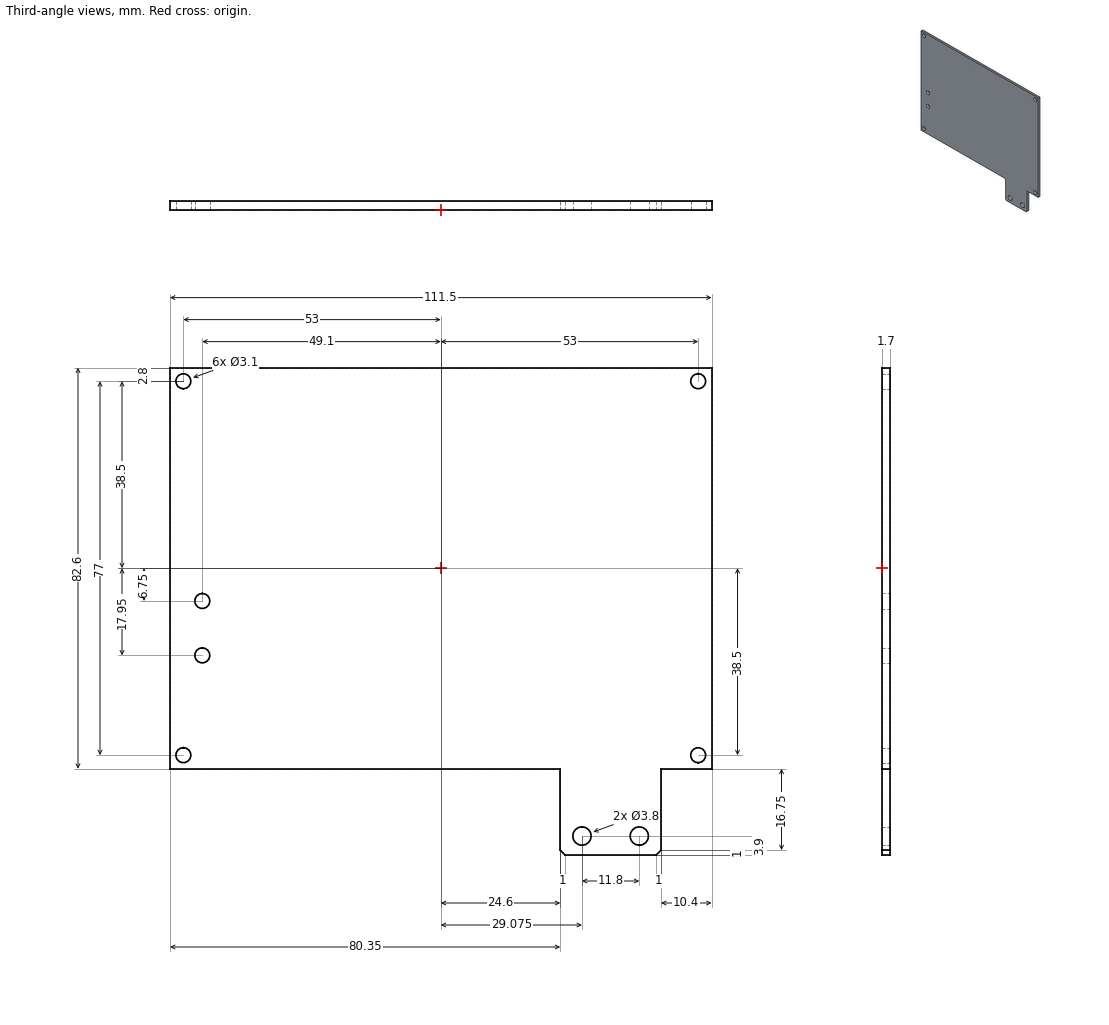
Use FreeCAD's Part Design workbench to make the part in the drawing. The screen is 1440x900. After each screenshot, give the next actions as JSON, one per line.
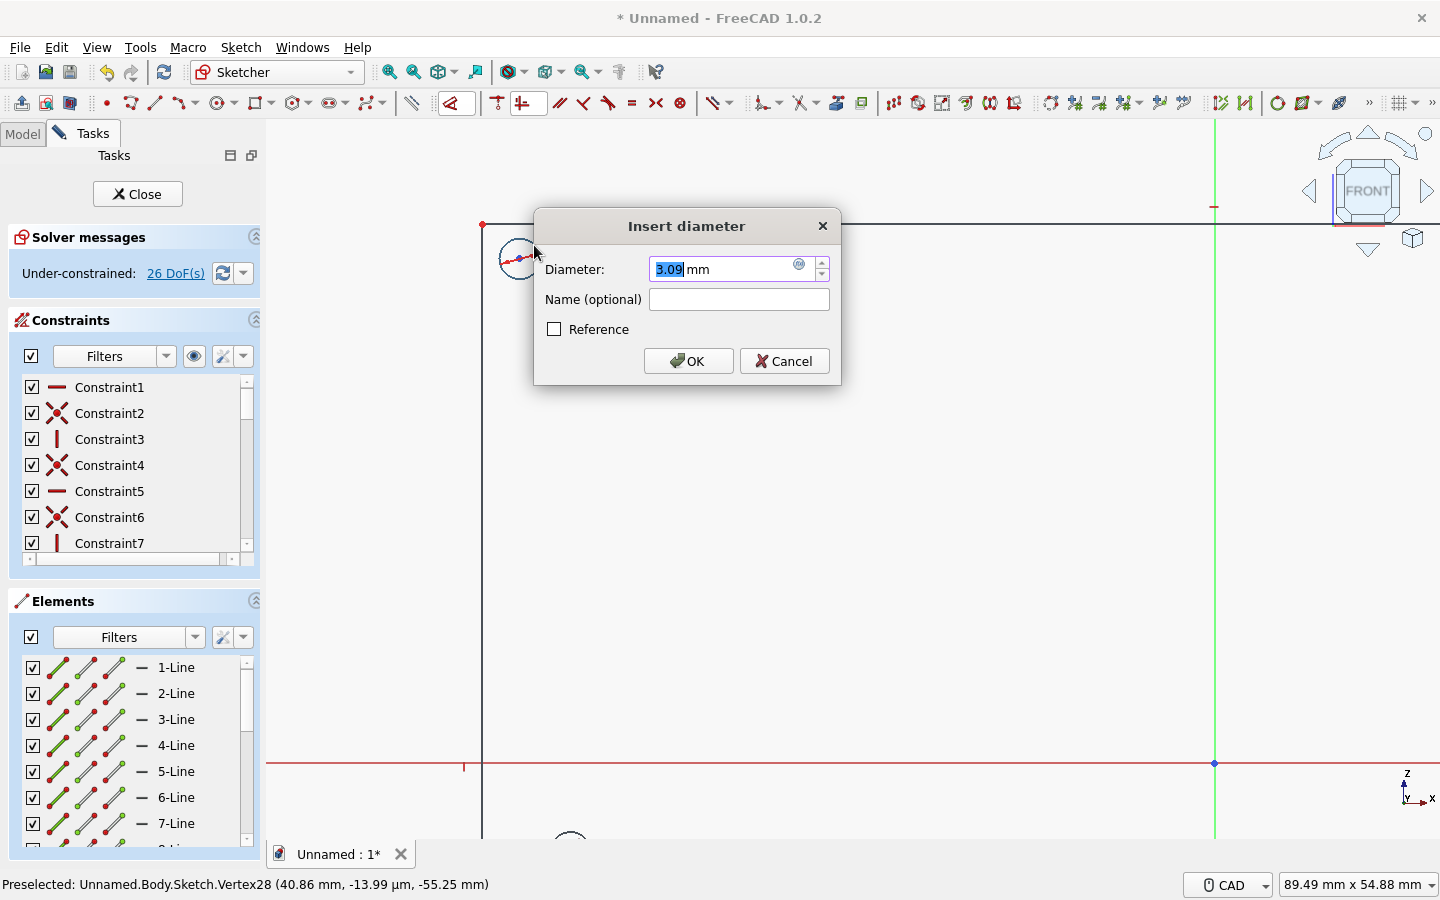
{"action": "type", "text": "3.1"}
{"action": "key", "text": "Return"}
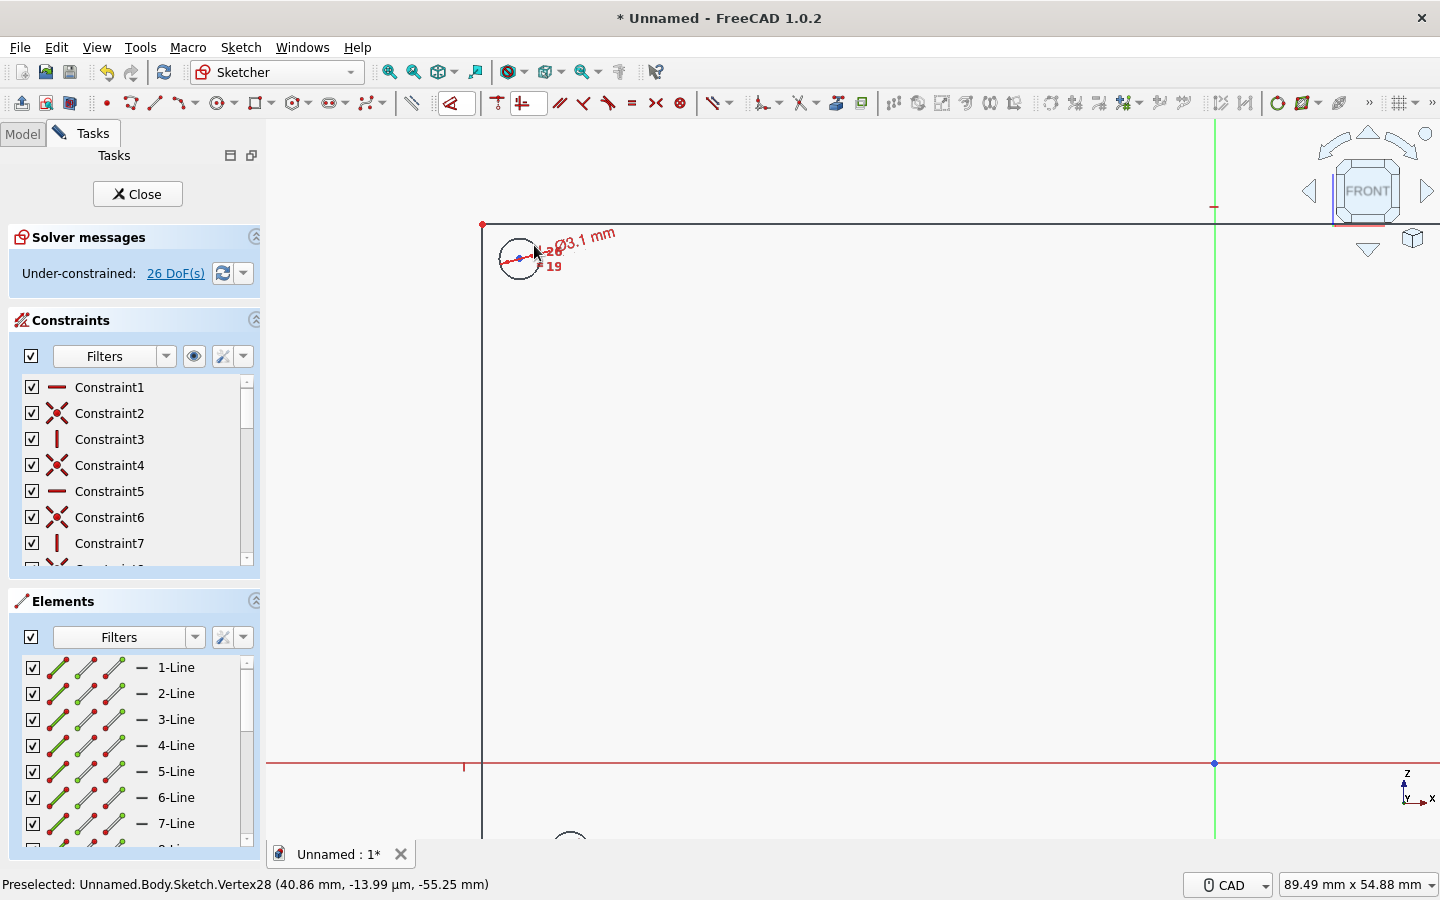
{"action": "scroll", "coordinate": [534, 246], "scroll_direction": "down", "scroll_amount": 5}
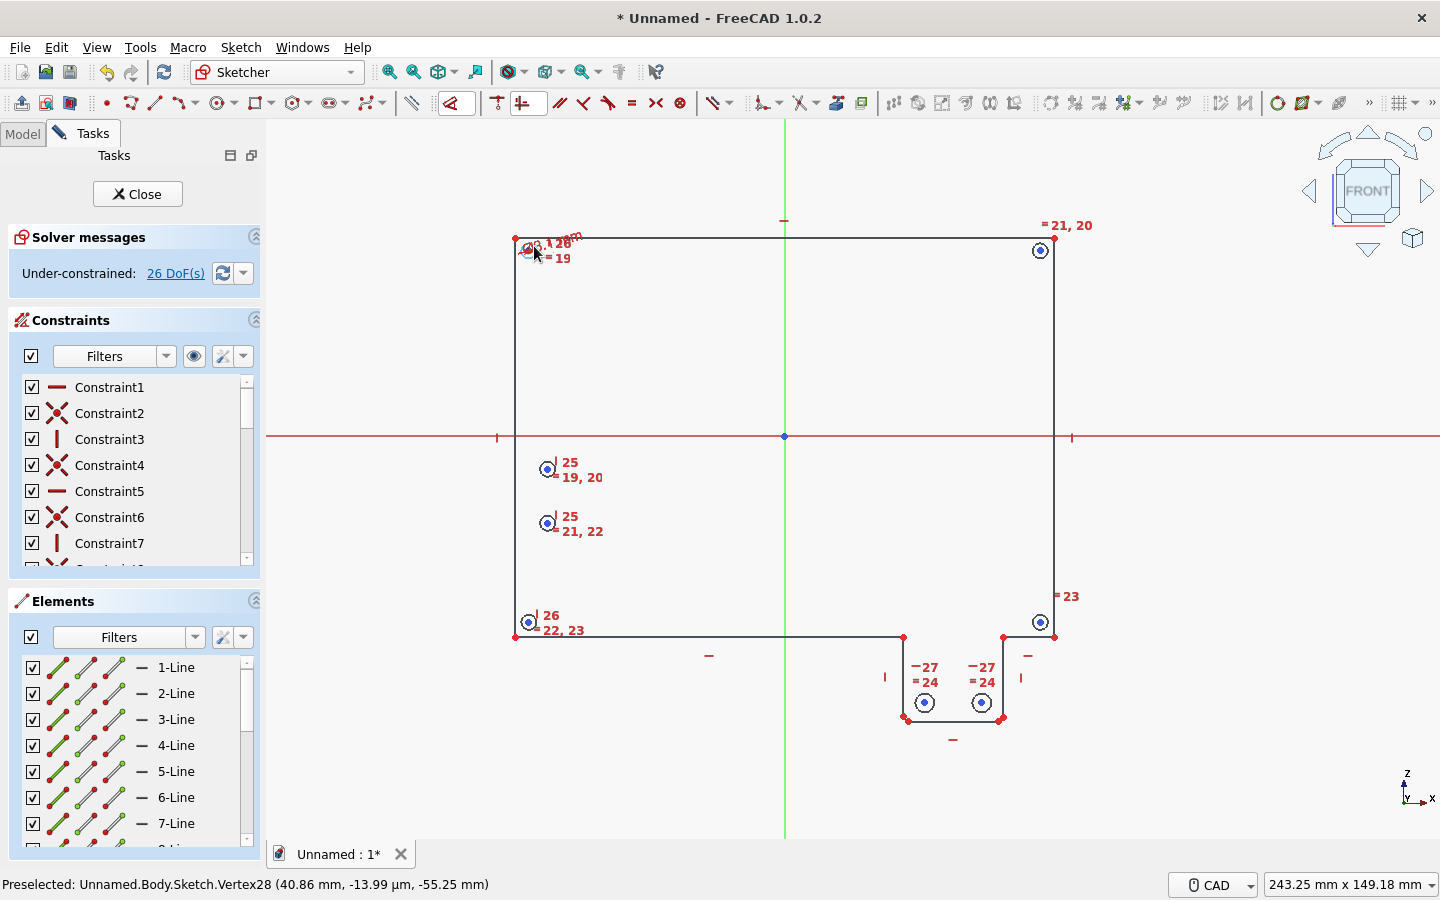
{"action": "scroll", "coordinate": [931, 696], "scroll_direction": "up", "scroll_amount": 4}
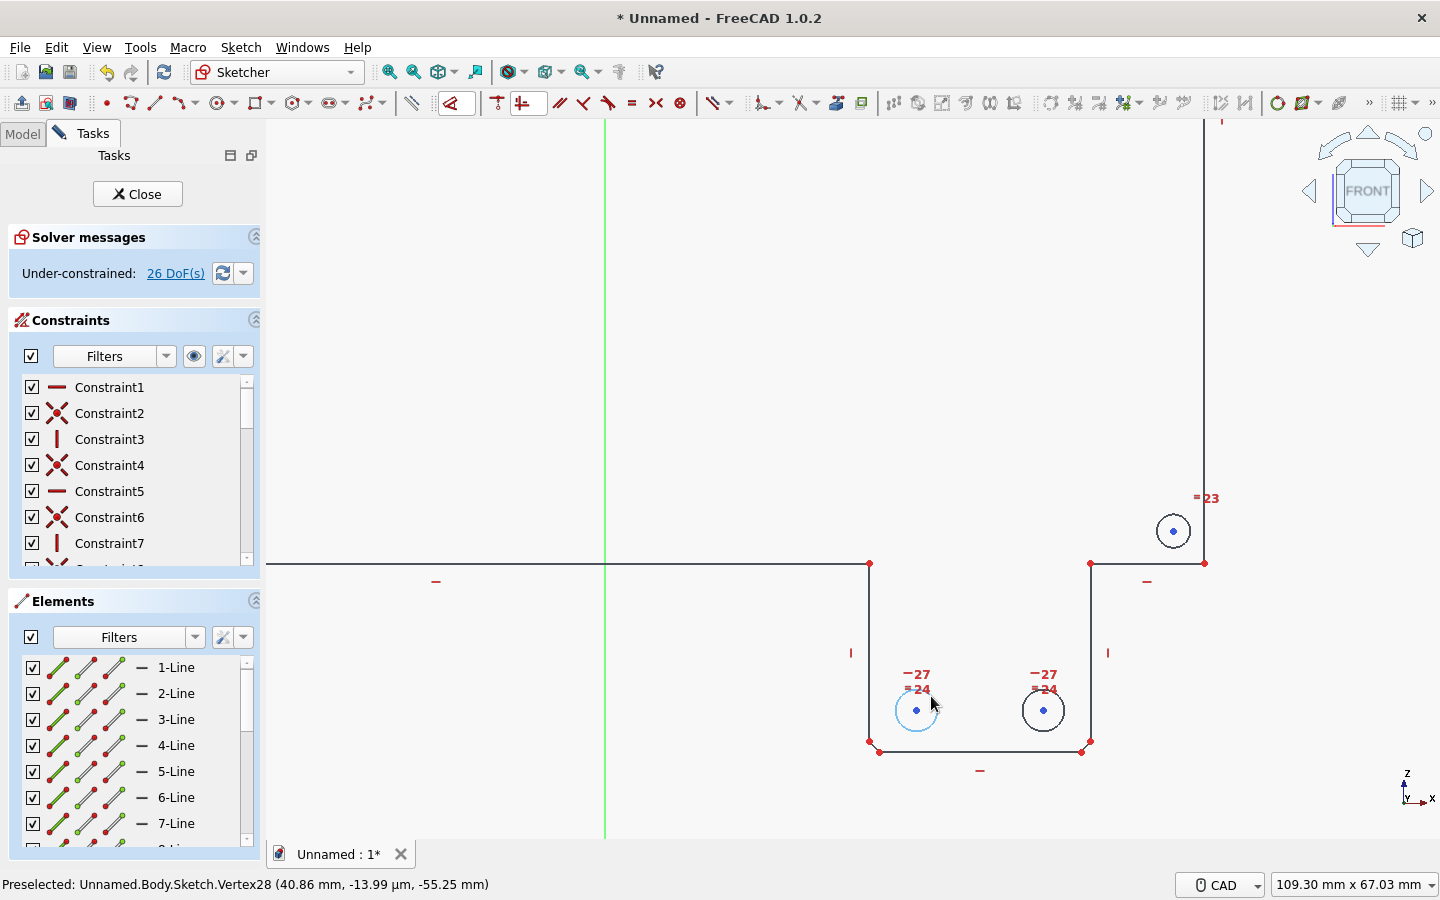
{"action": "left_click", "coordinate": [931, 696]}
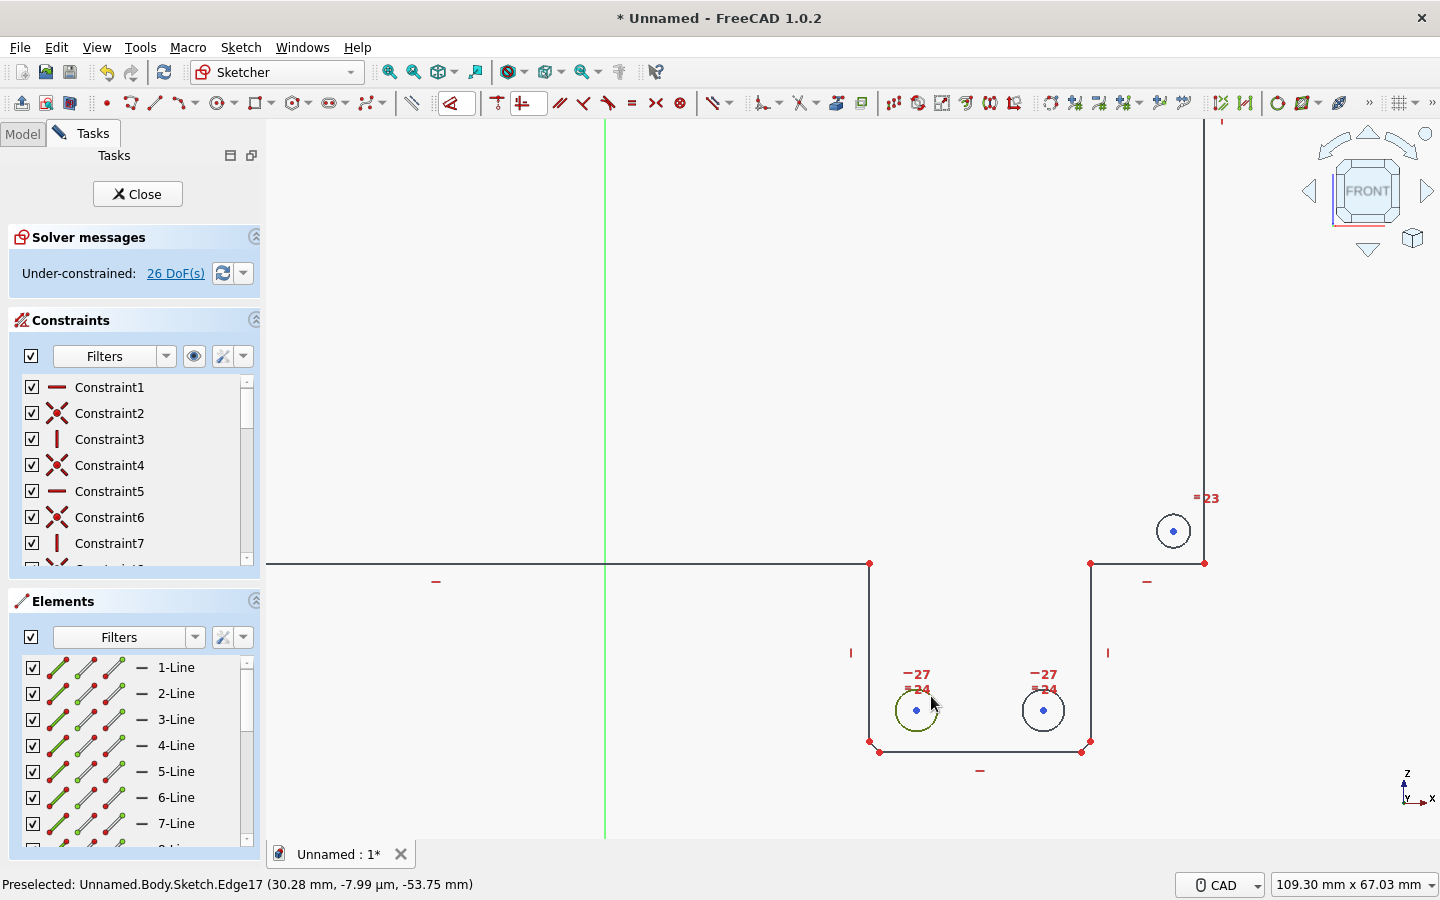
{"action": "left_click", "coordinate": [470, 104]}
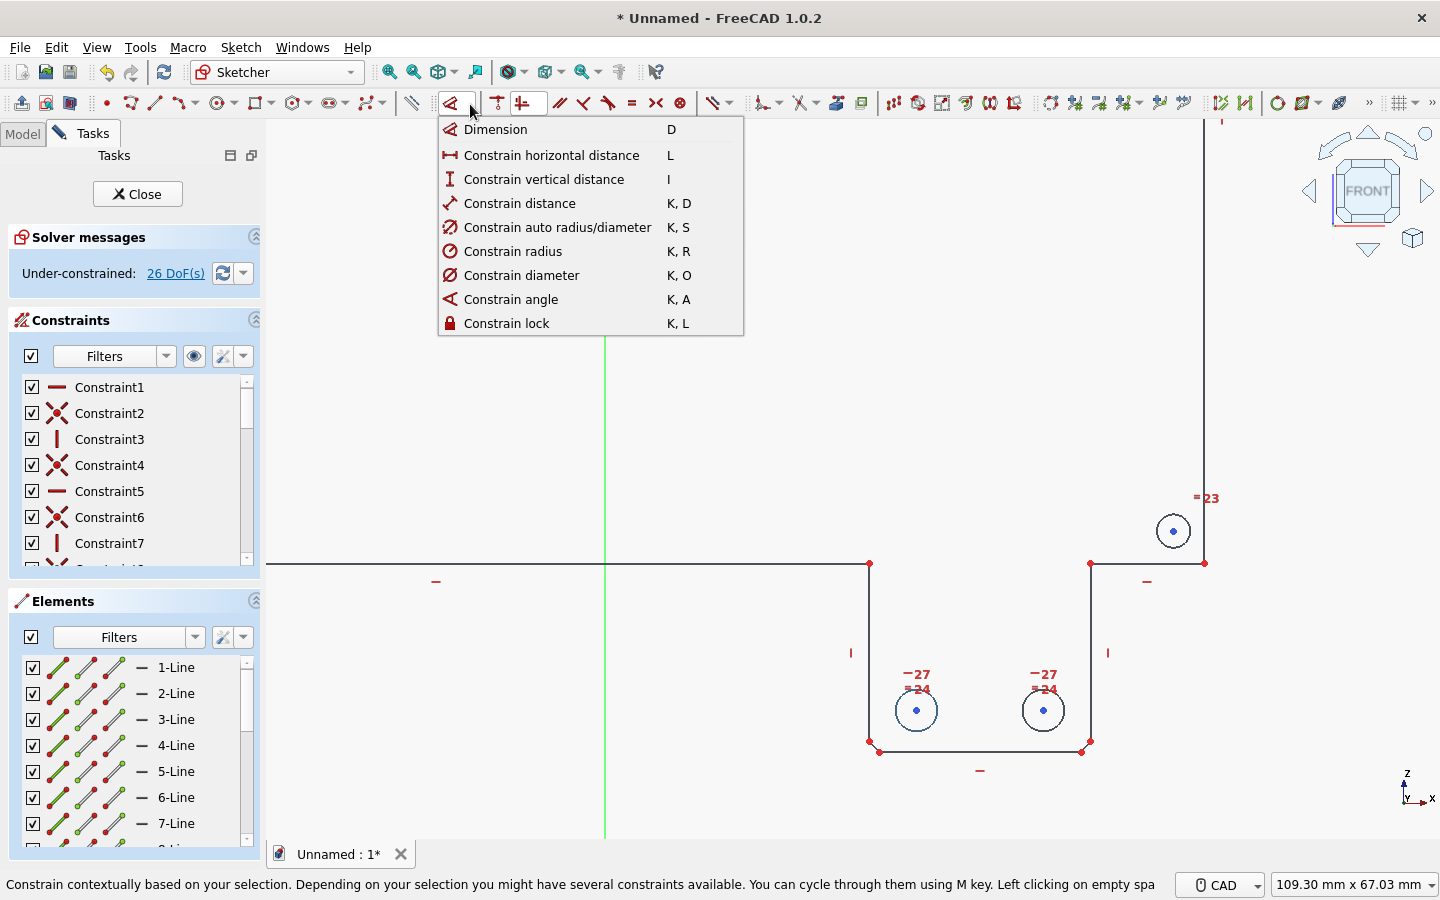
{"action": "left_click", "coordinate": [591, 275]}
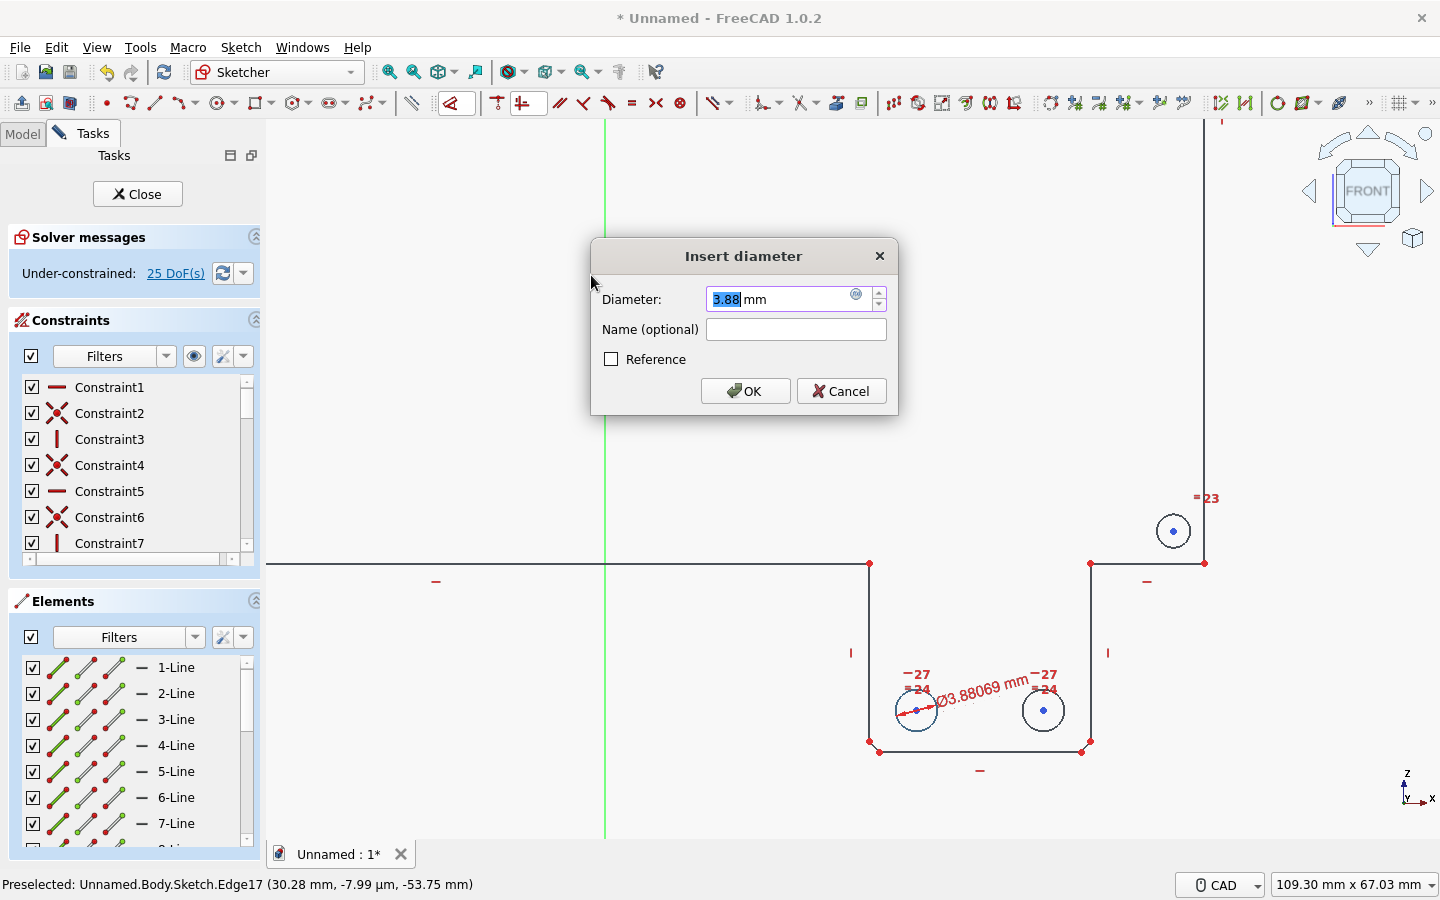
{"action": "type", "text": "3.8"}
{"action": "key", "text": "Return"}